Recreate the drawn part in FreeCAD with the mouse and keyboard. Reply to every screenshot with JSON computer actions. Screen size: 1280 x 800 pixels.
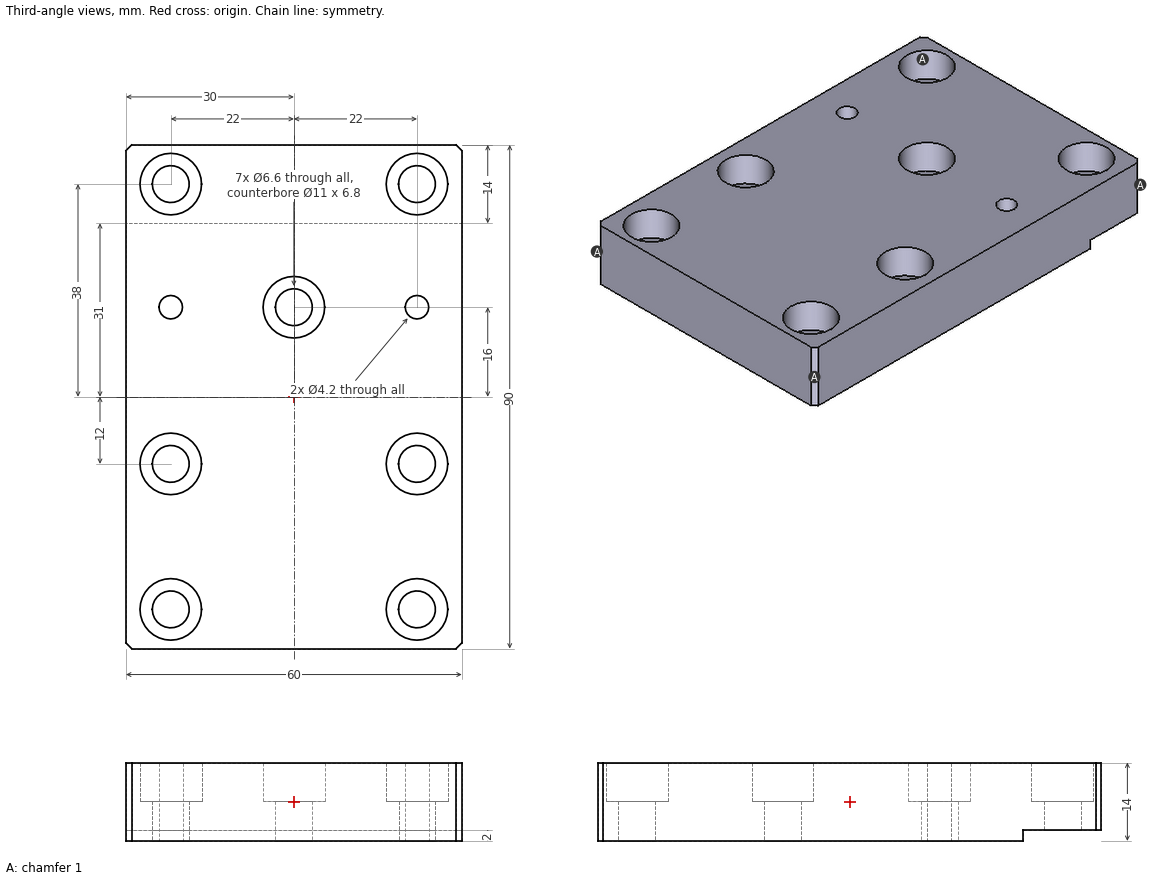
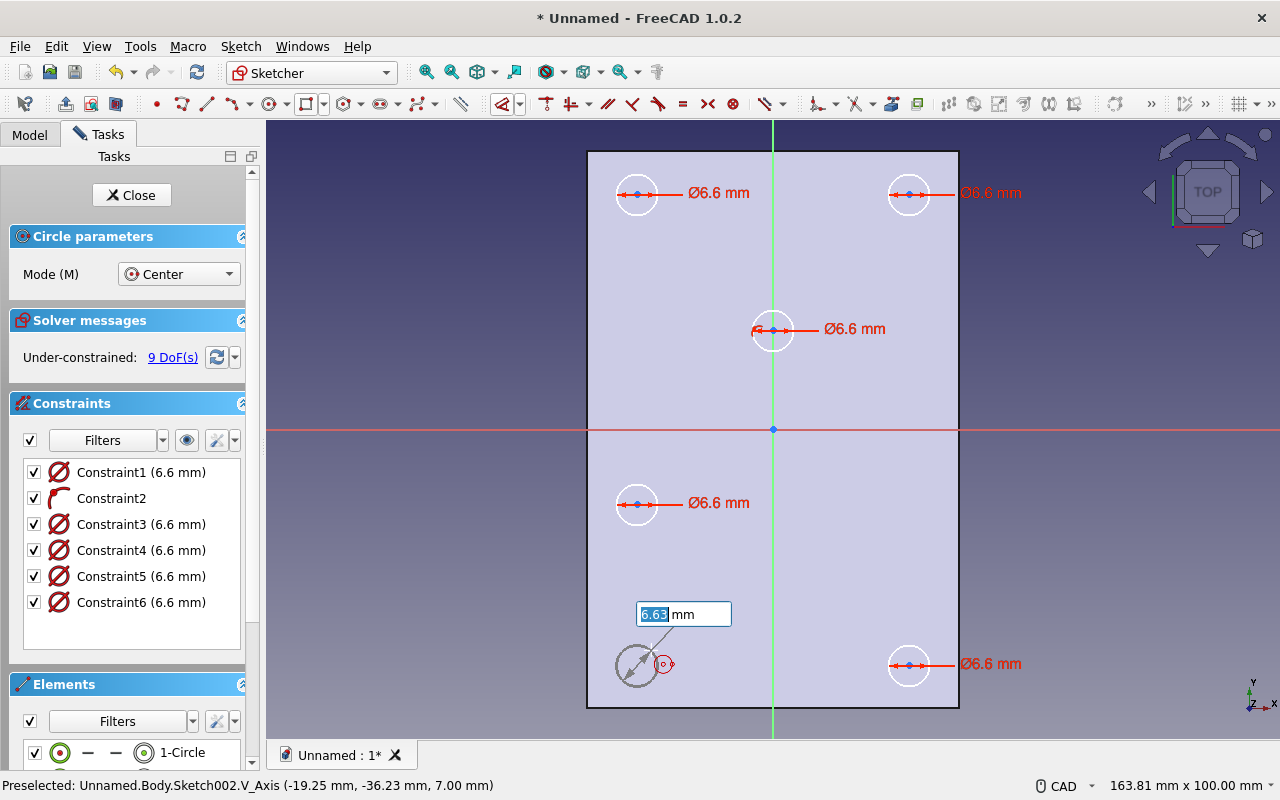
{"action": "type", "text": "6.6"}
{"action": "key", "text": "Return"}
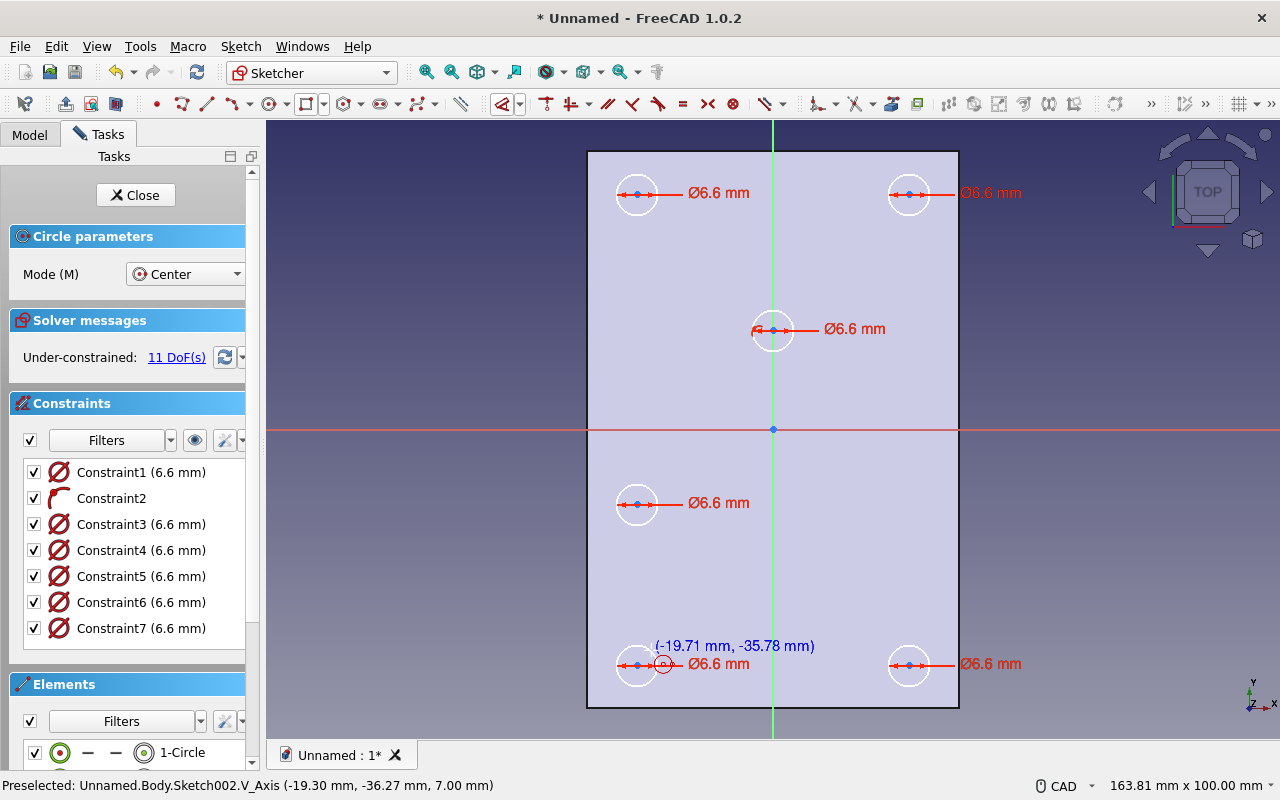
{"action": "left_click", "coordinate": [909, 504]}
{"action": "mouse_move", "coordinate": [924, 489]}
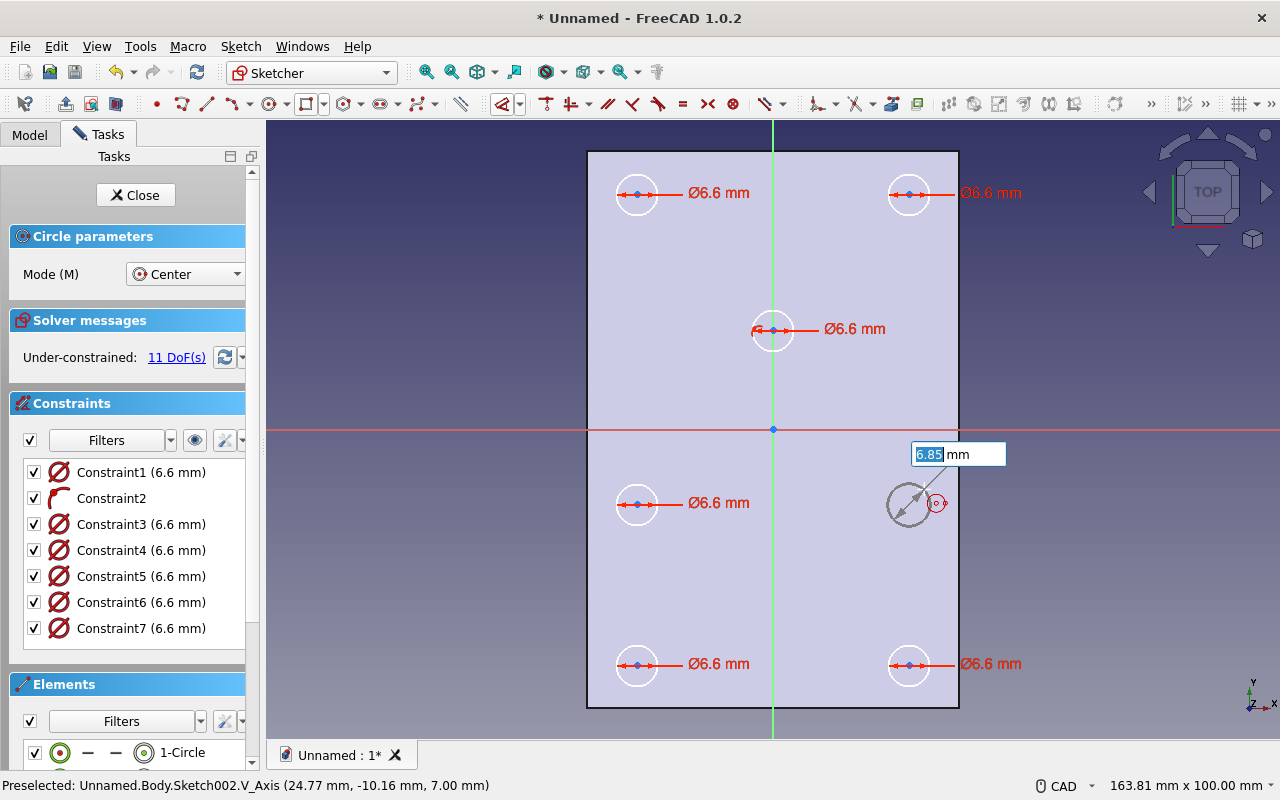
{"action": "type", "text": "6.6"}
{"action": "key", "text": "Return"}
{"action": "key", "text": "Escape"}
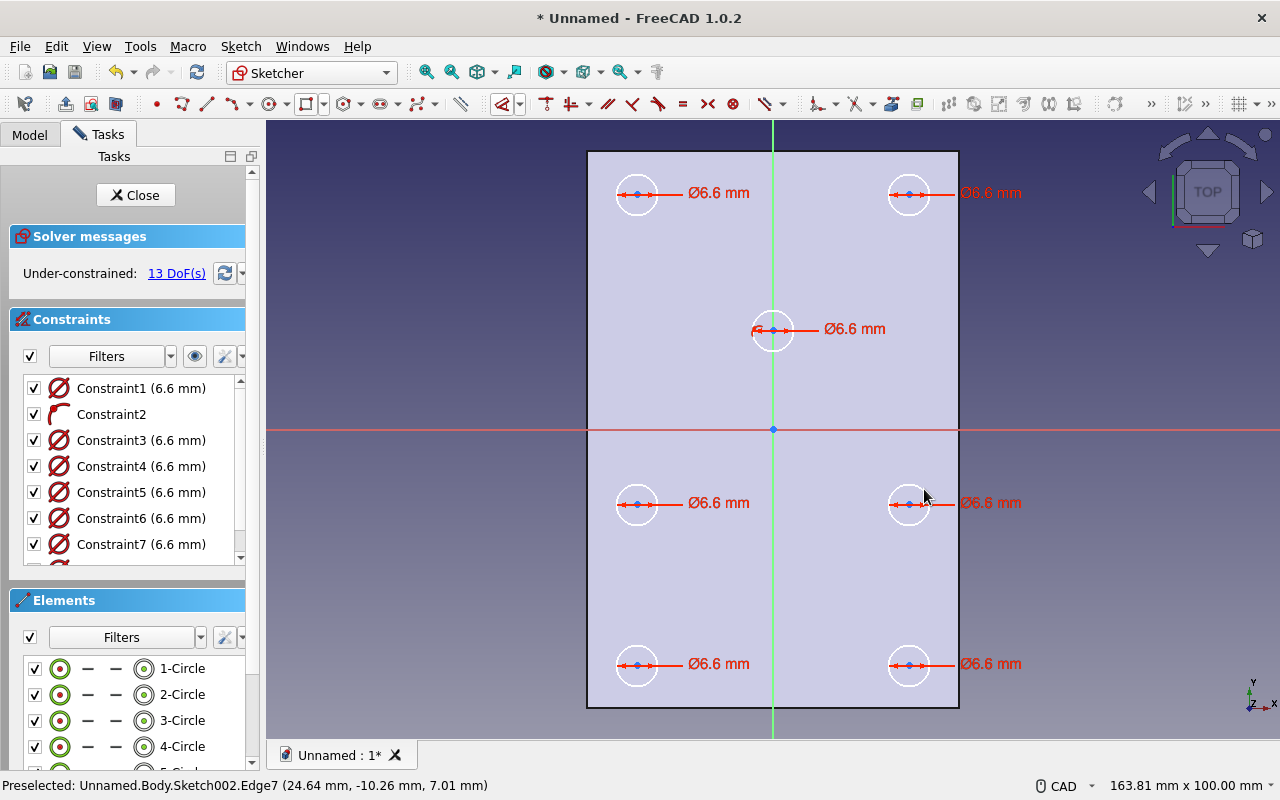
{"action": "left_click", "coordinate": [637, 195]}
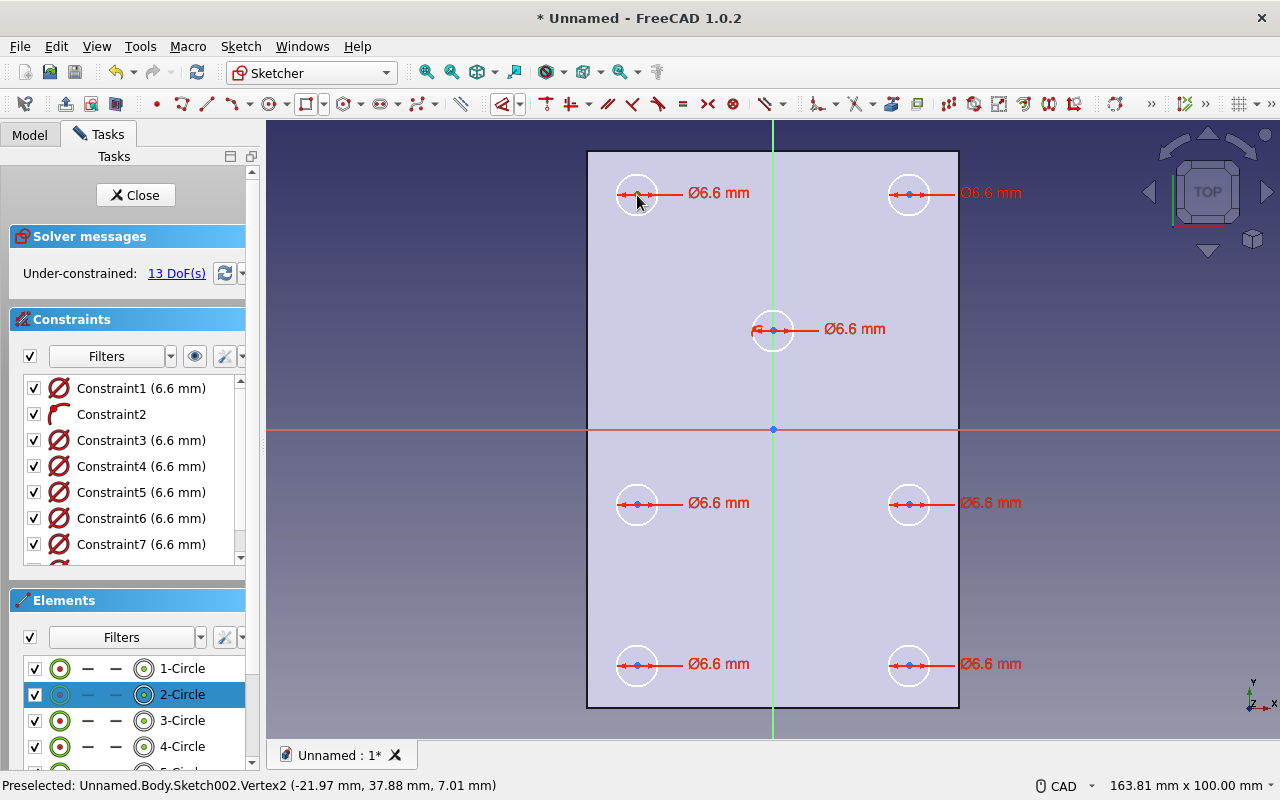
{"action": "left_click", "coordinate": [909, 195]}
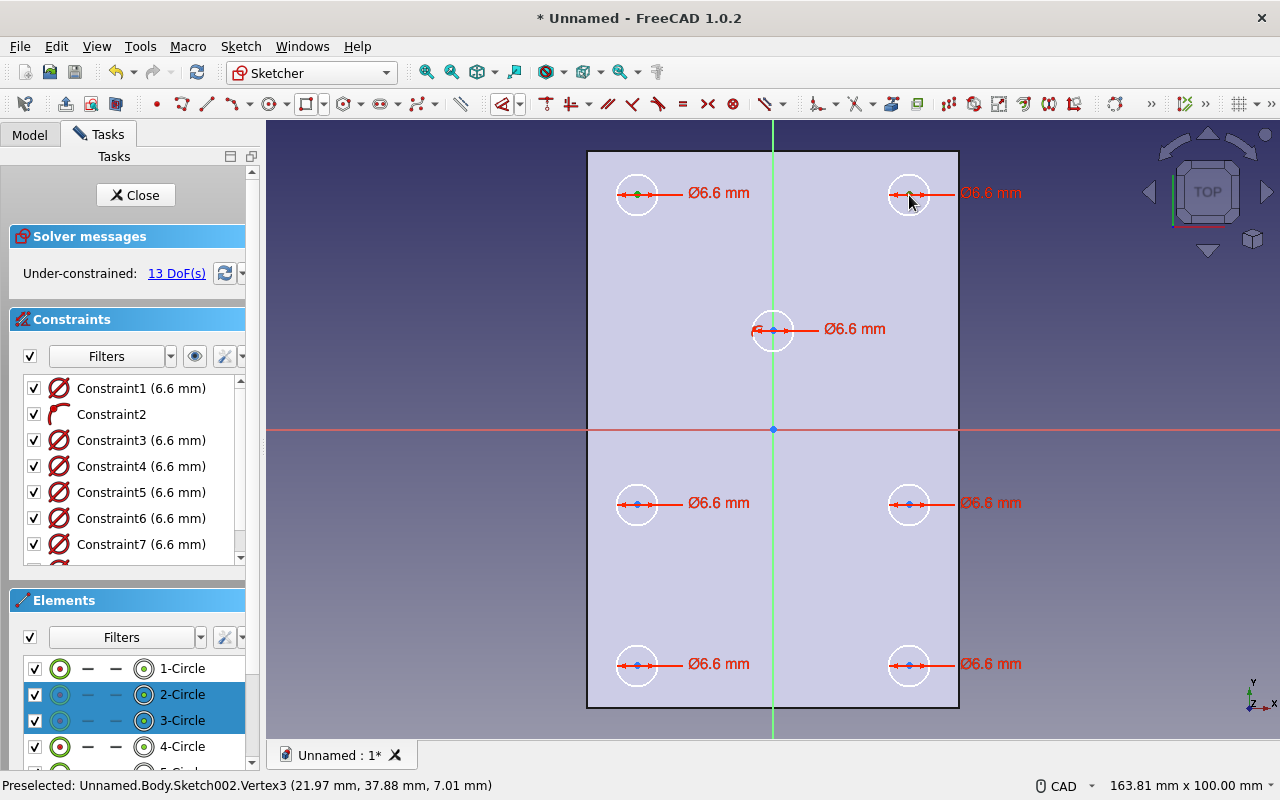
{"action": "left_click", "coordinate": [773, 671]}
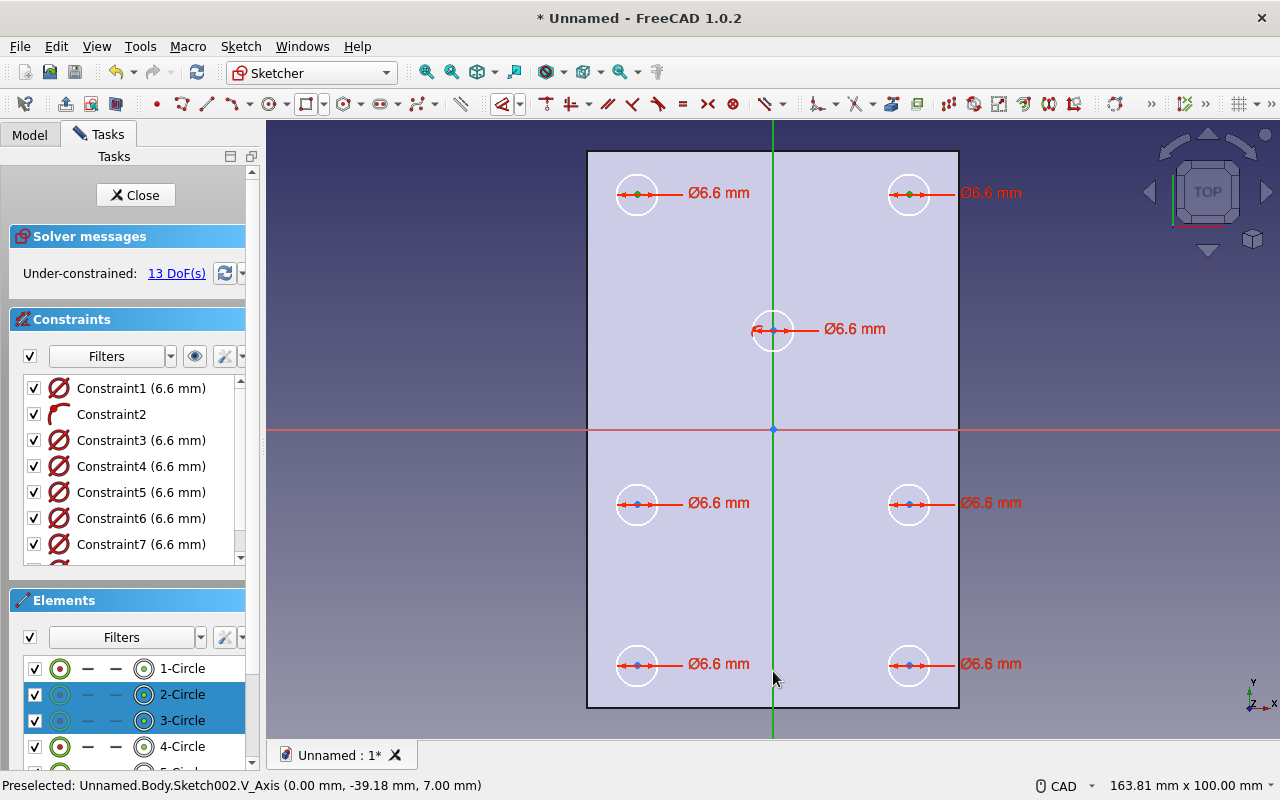
{"action": "left_click", "coordinate": [708, 104]}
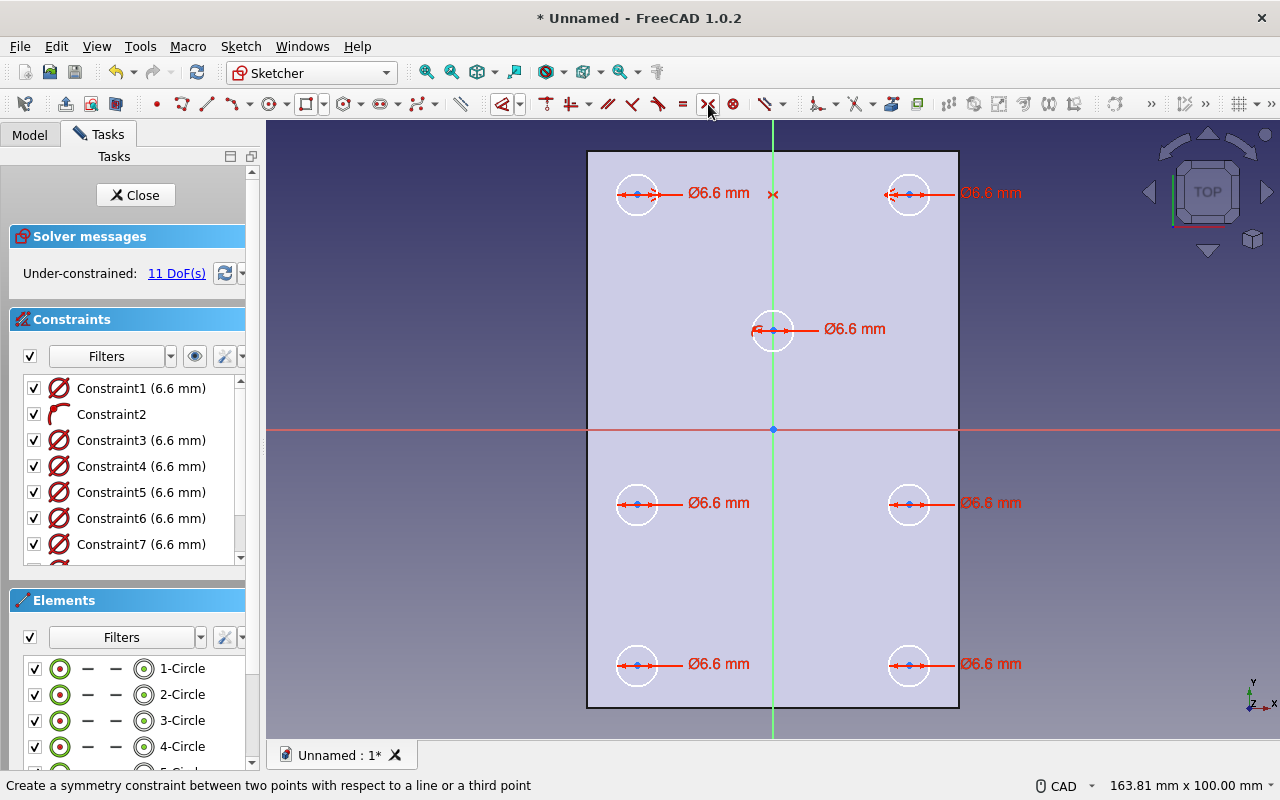
{"action": "left_click", "coordinate": [909, 195]}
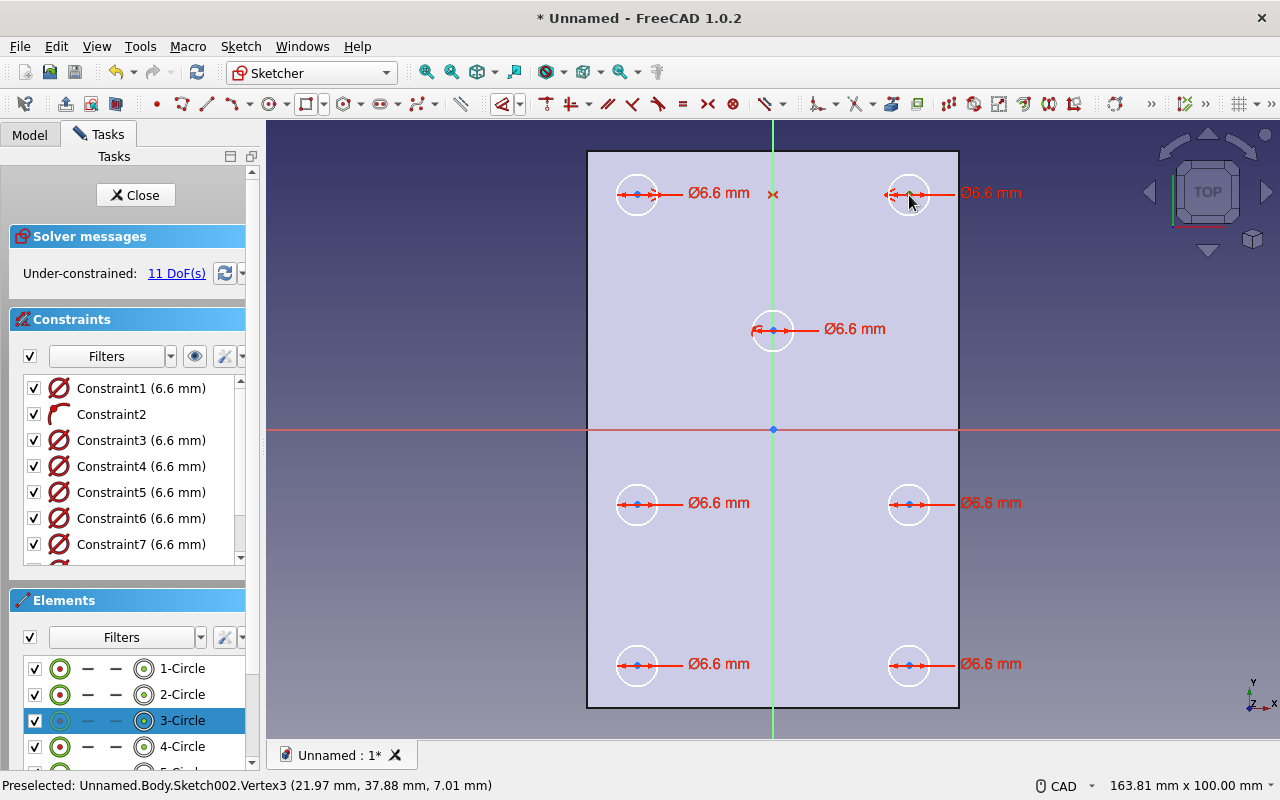
{"action": "left_click", "coordinate": [909, 666]}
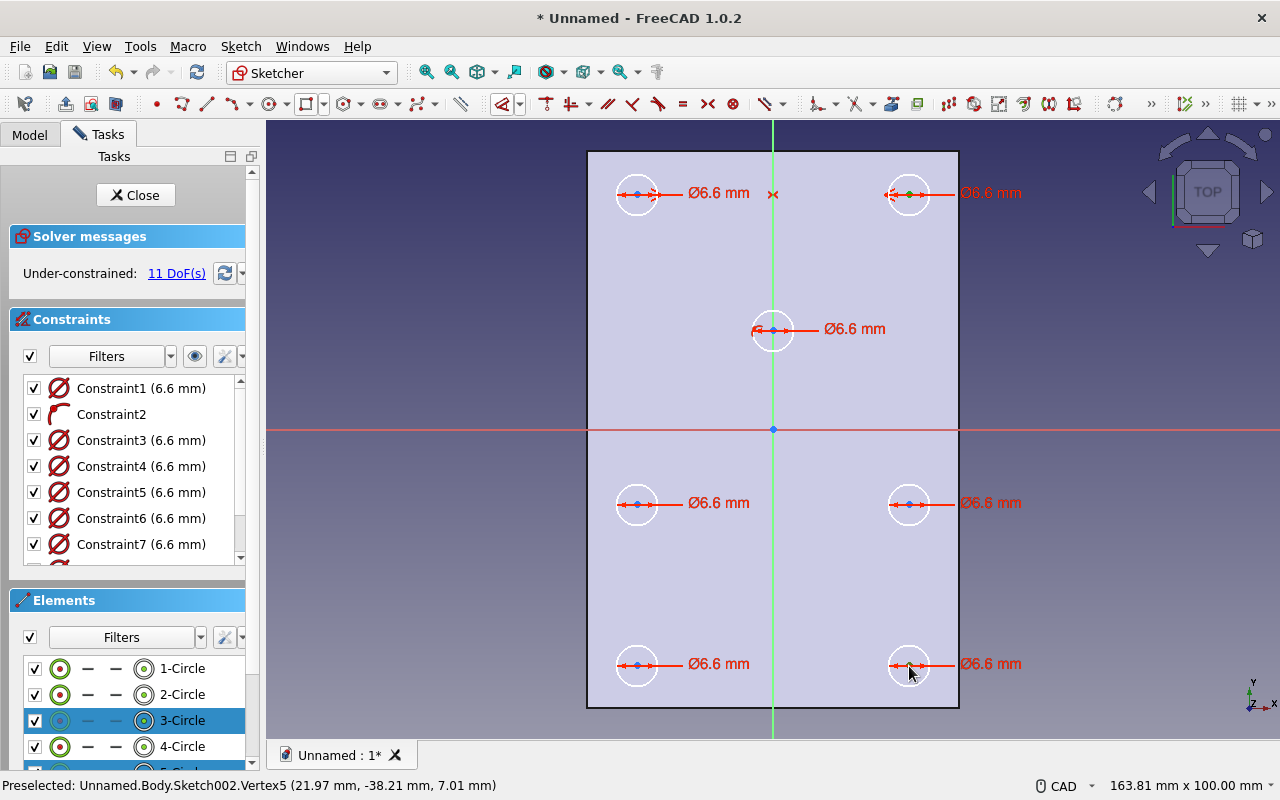
{"action": "left_click", "coordinate": [353, 429]}